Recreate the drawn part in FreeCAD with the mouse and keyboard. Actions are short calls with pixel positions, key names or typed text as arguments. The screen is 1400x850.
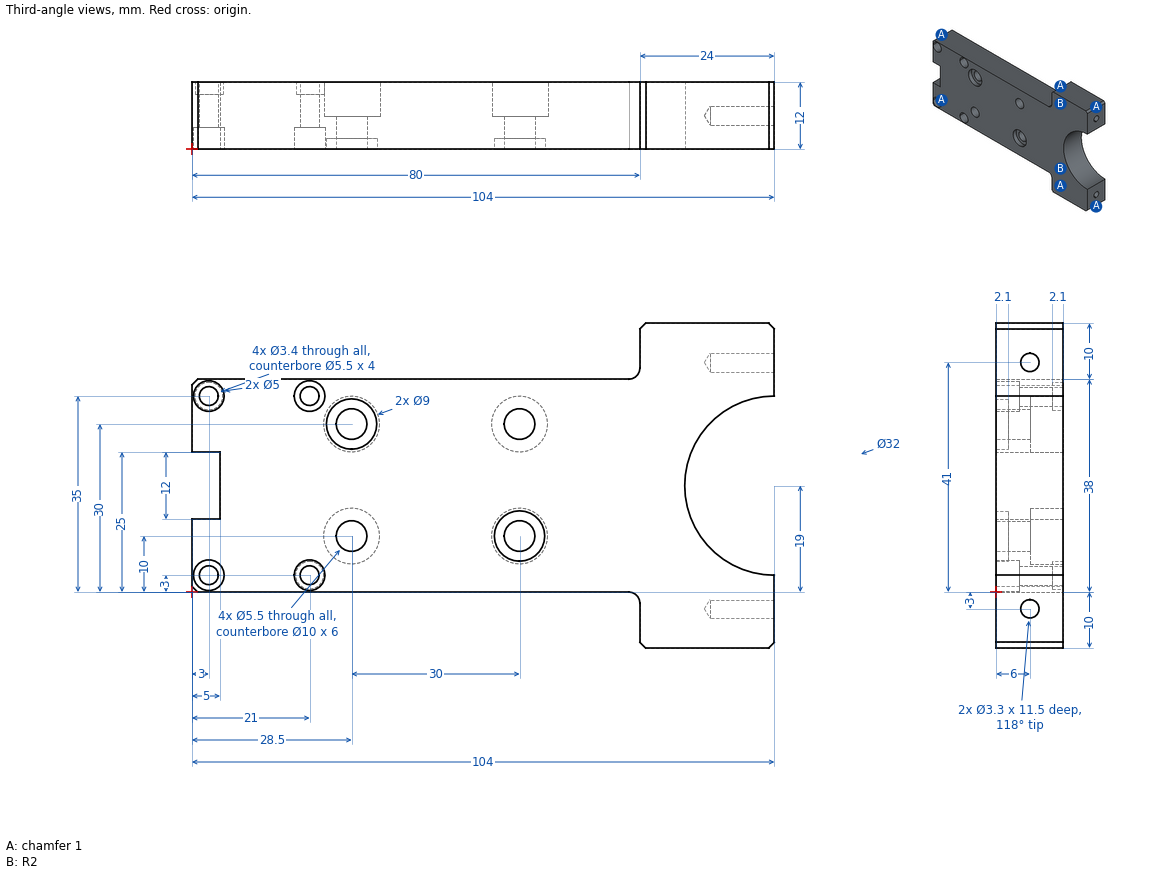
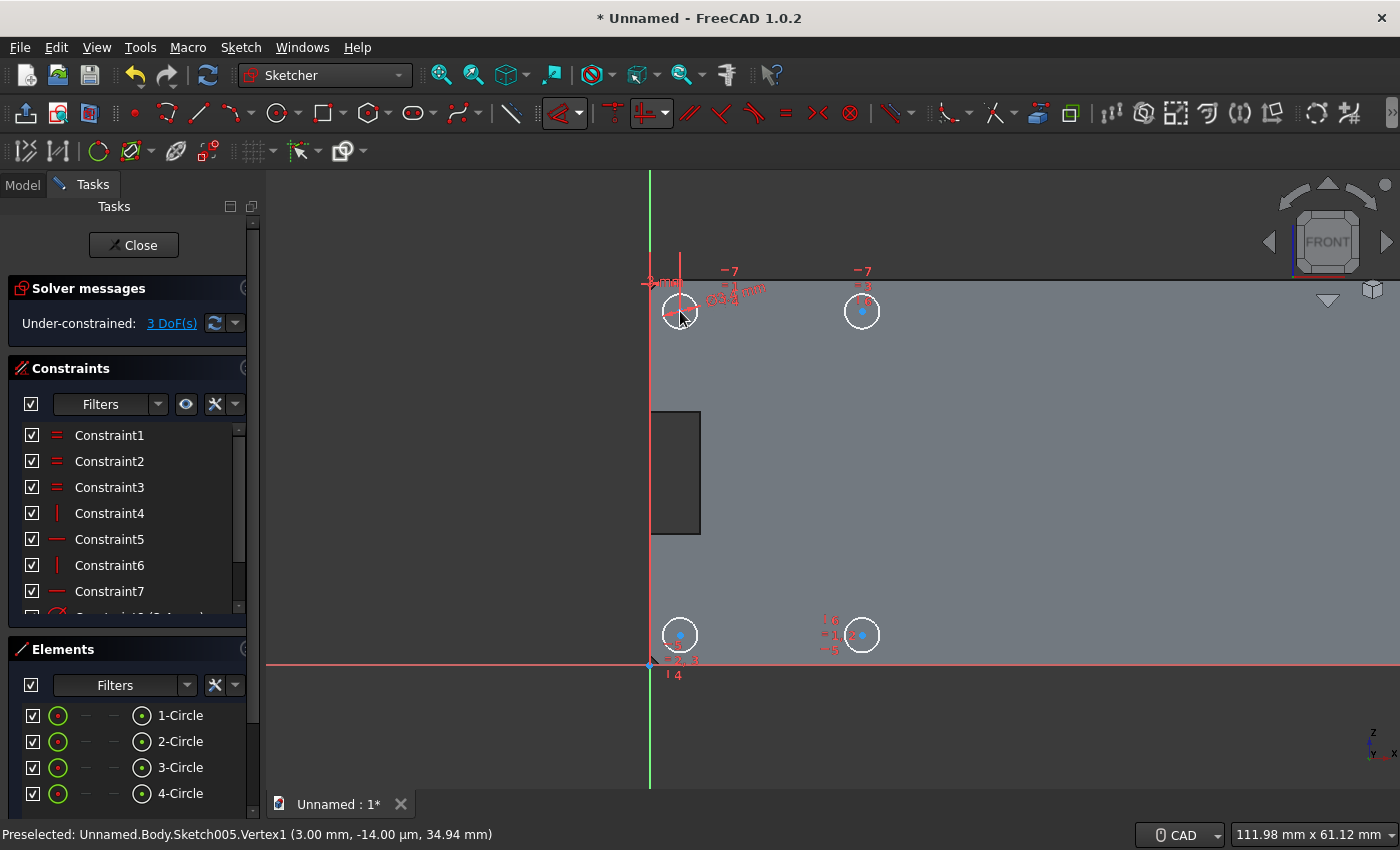
scroll(862, 635, up, 2)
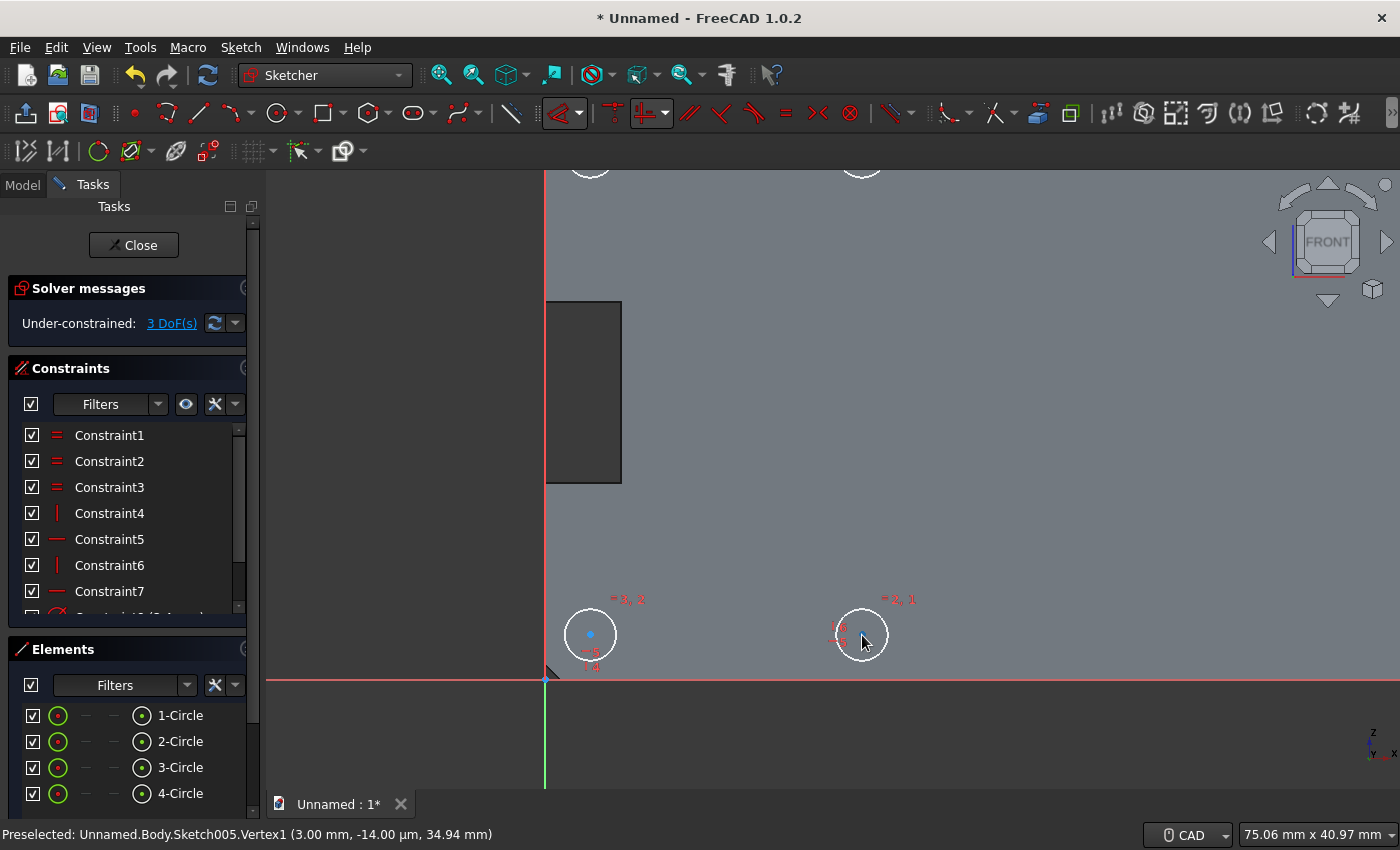
click(862, 635)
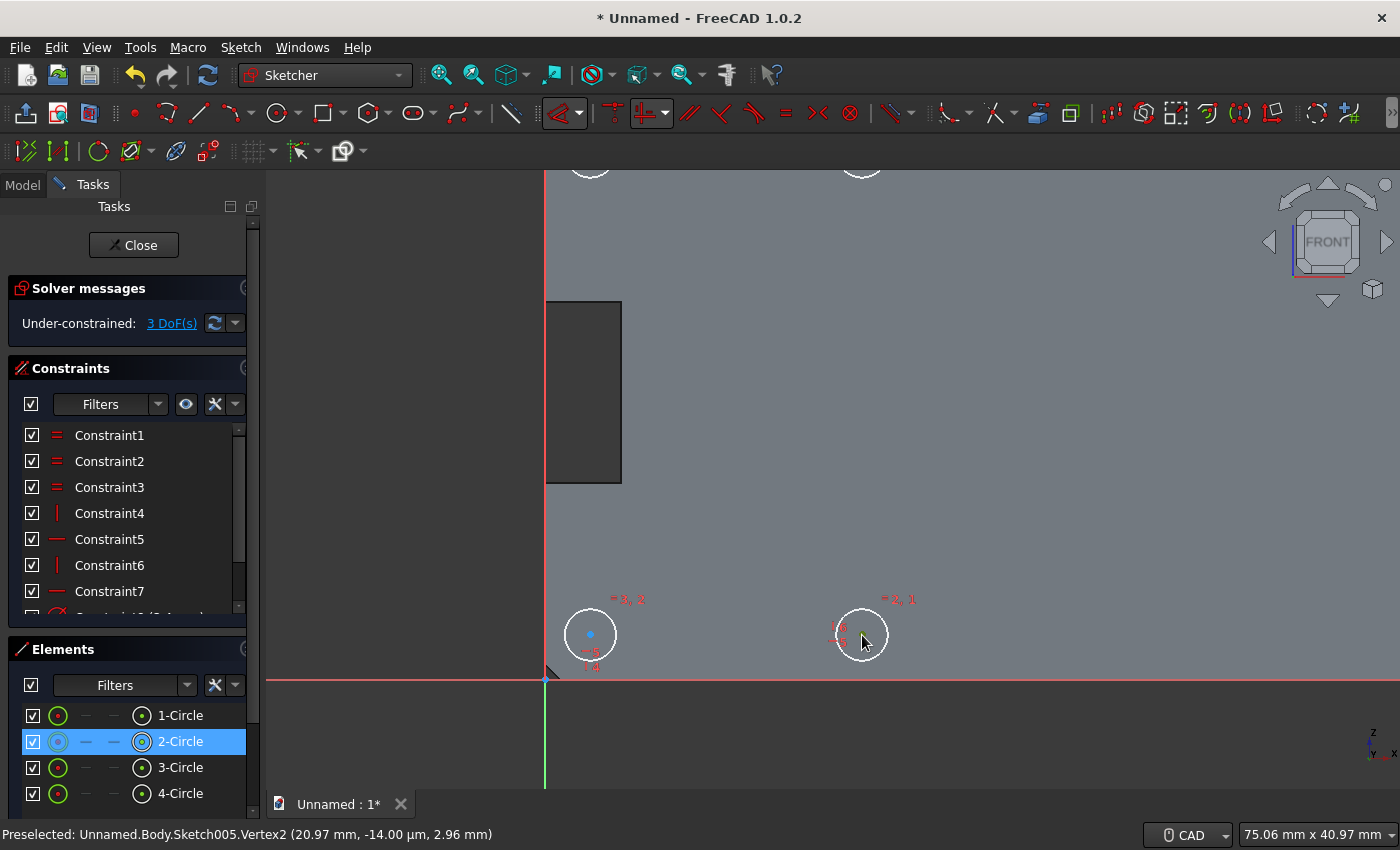
click(582, 114)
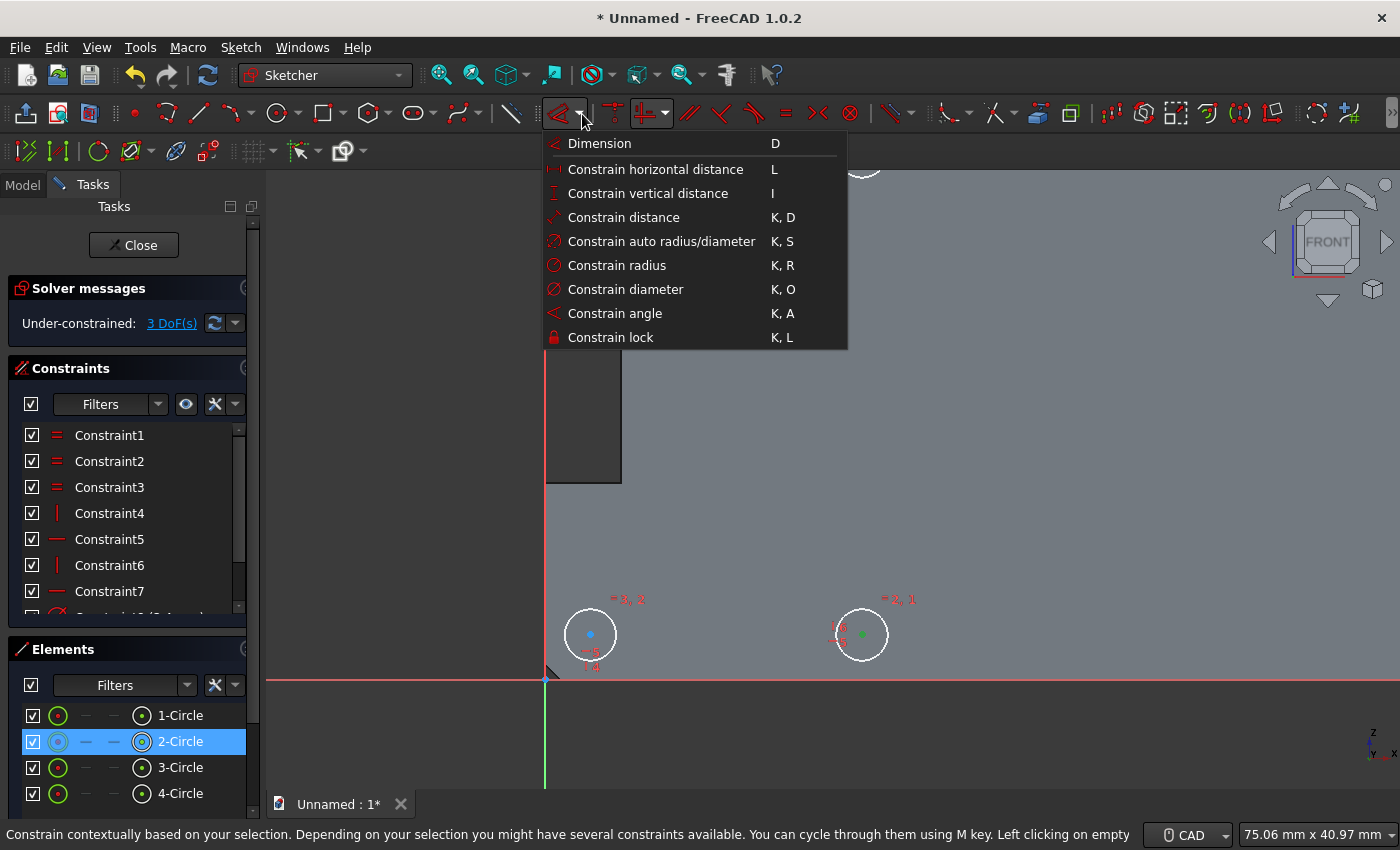
click(695, 193)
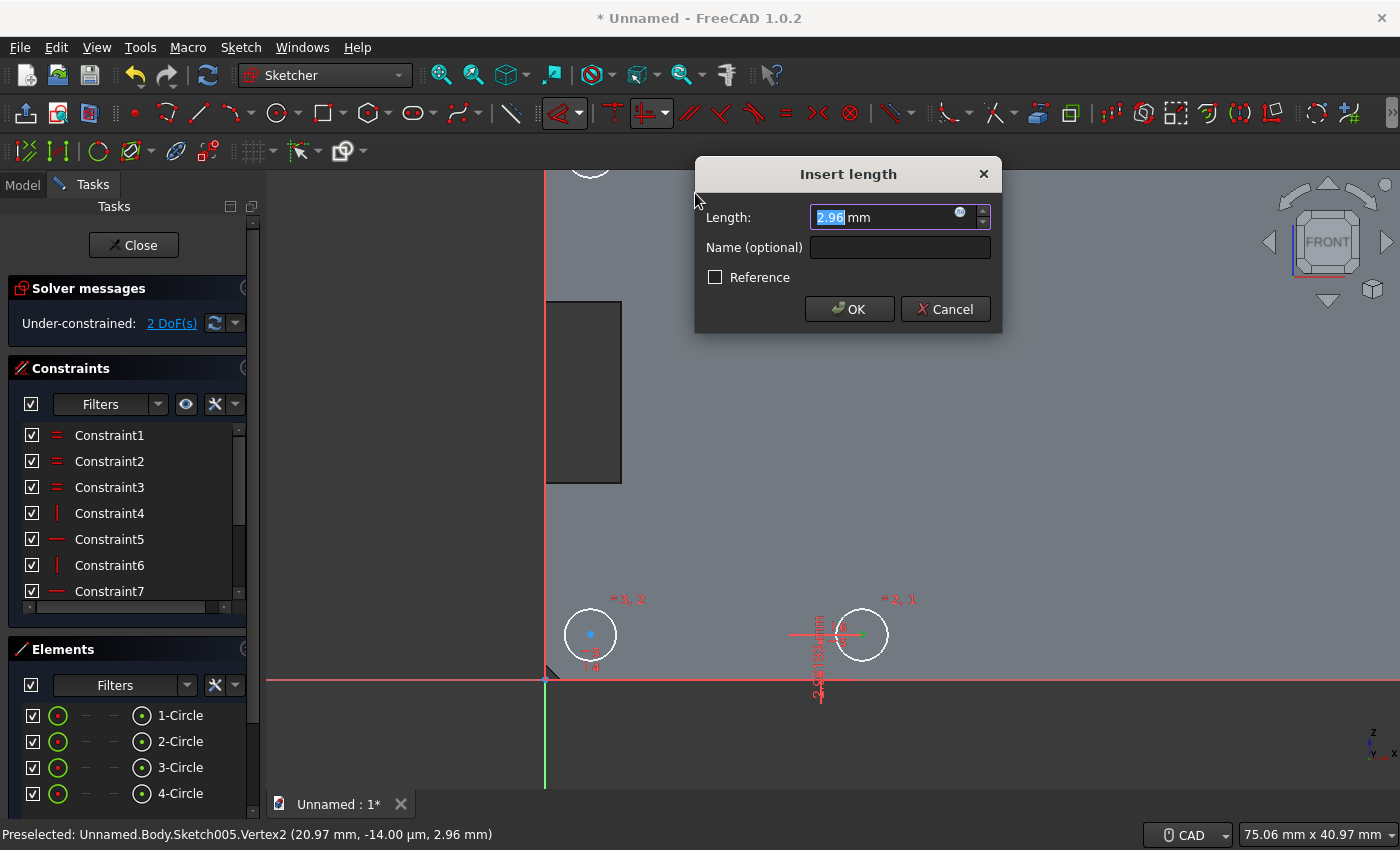
text(3)
key(Return)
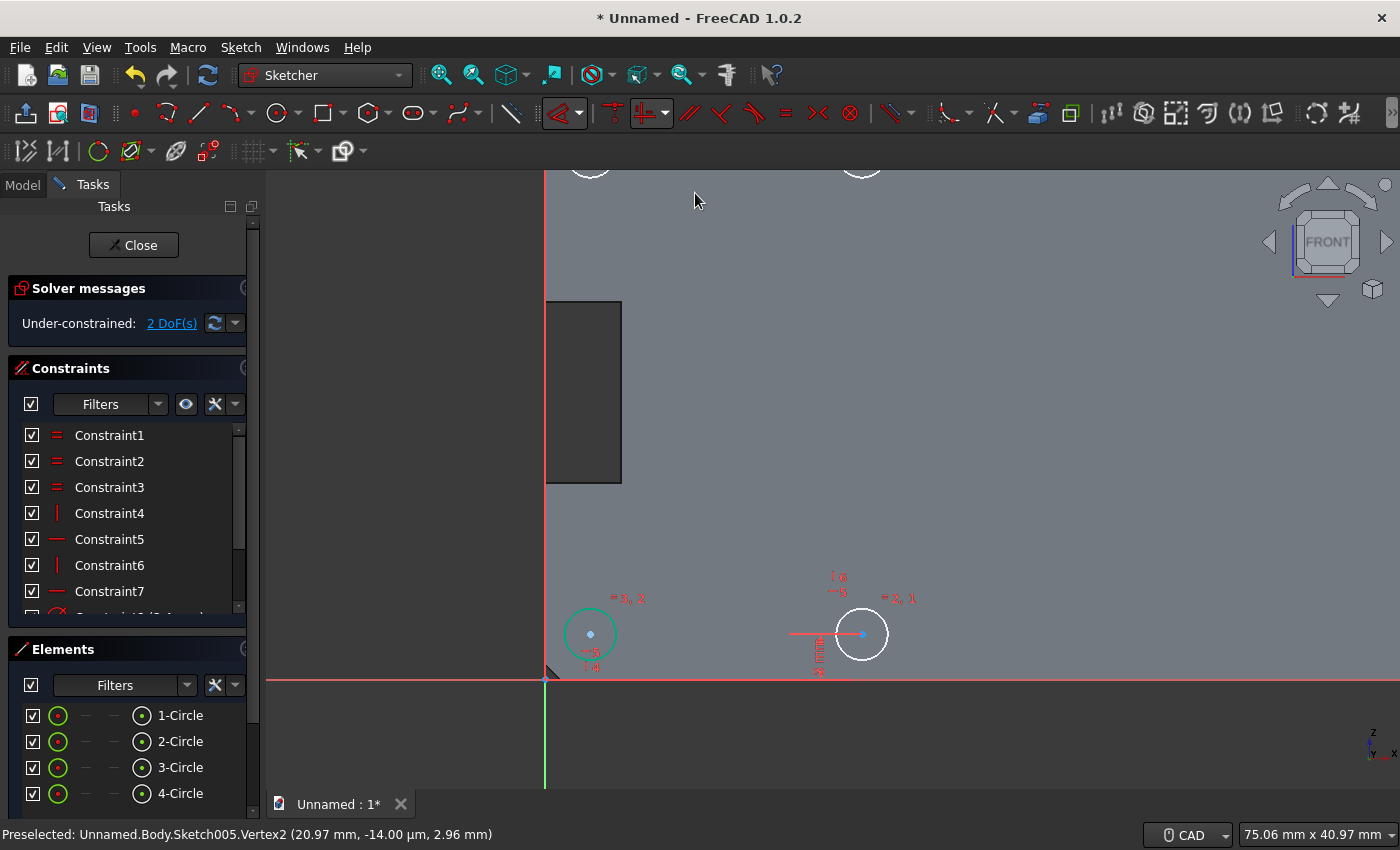
scroll(862, 636, down, 2)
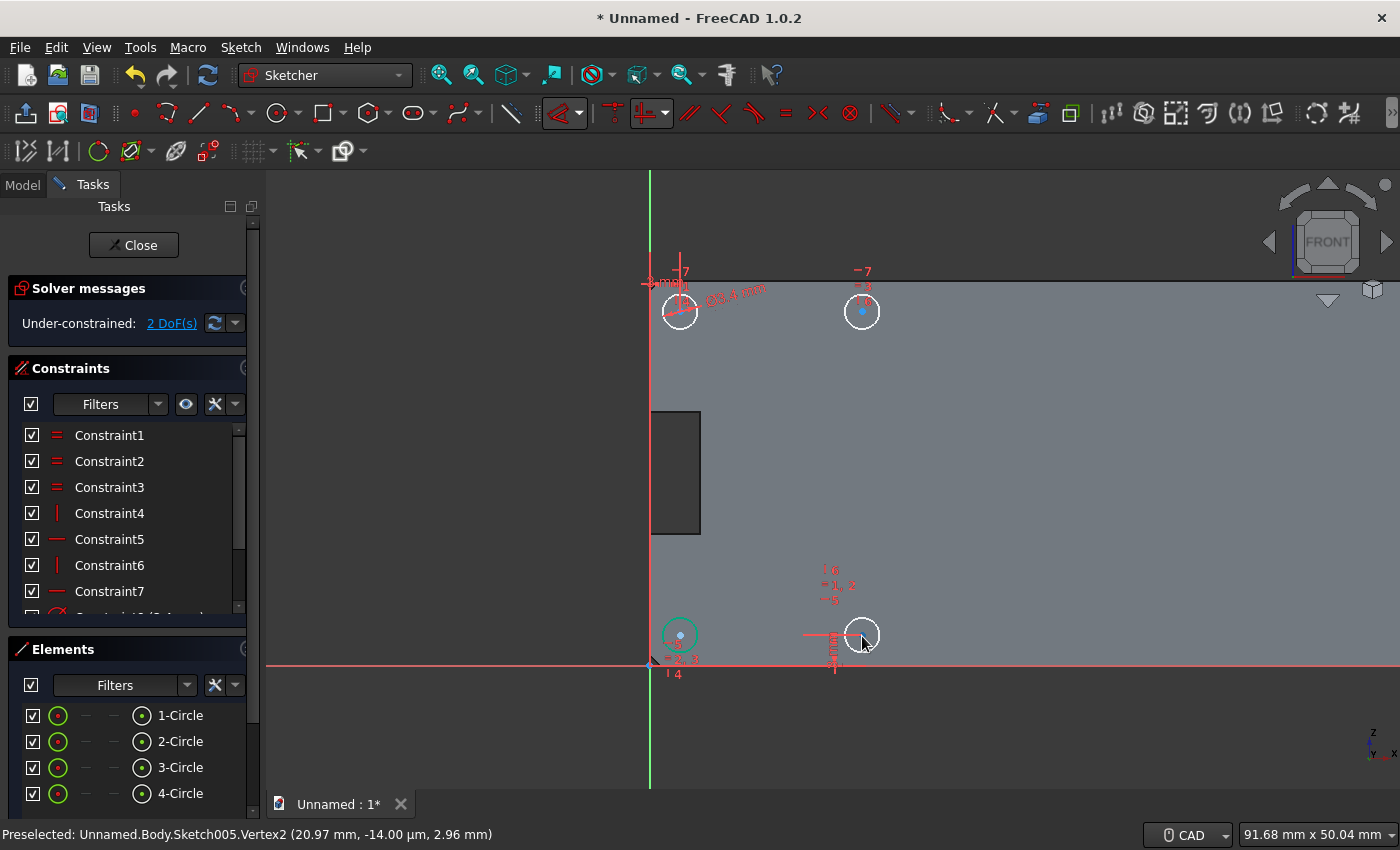
click(680, 312)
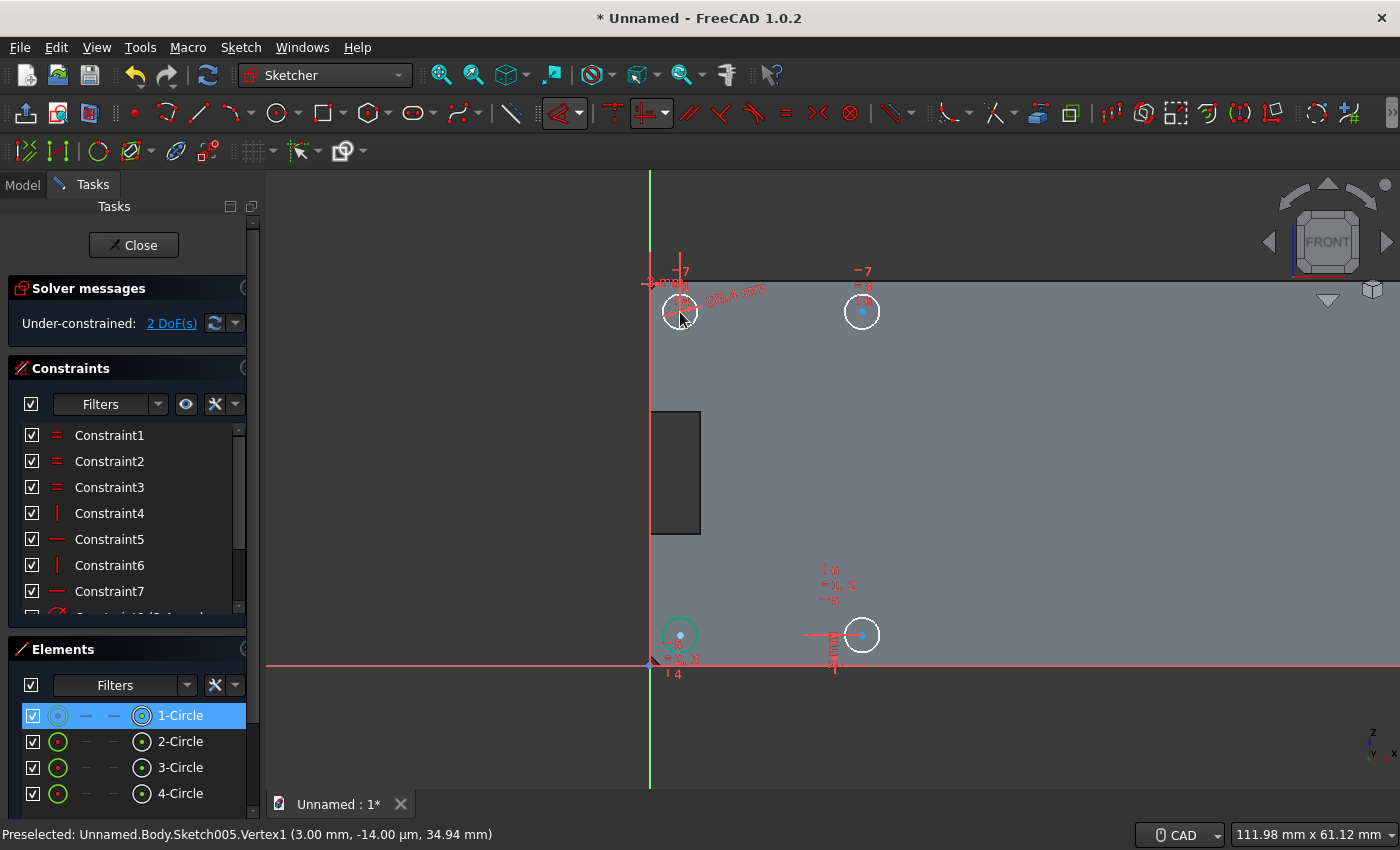
click(582, 114)